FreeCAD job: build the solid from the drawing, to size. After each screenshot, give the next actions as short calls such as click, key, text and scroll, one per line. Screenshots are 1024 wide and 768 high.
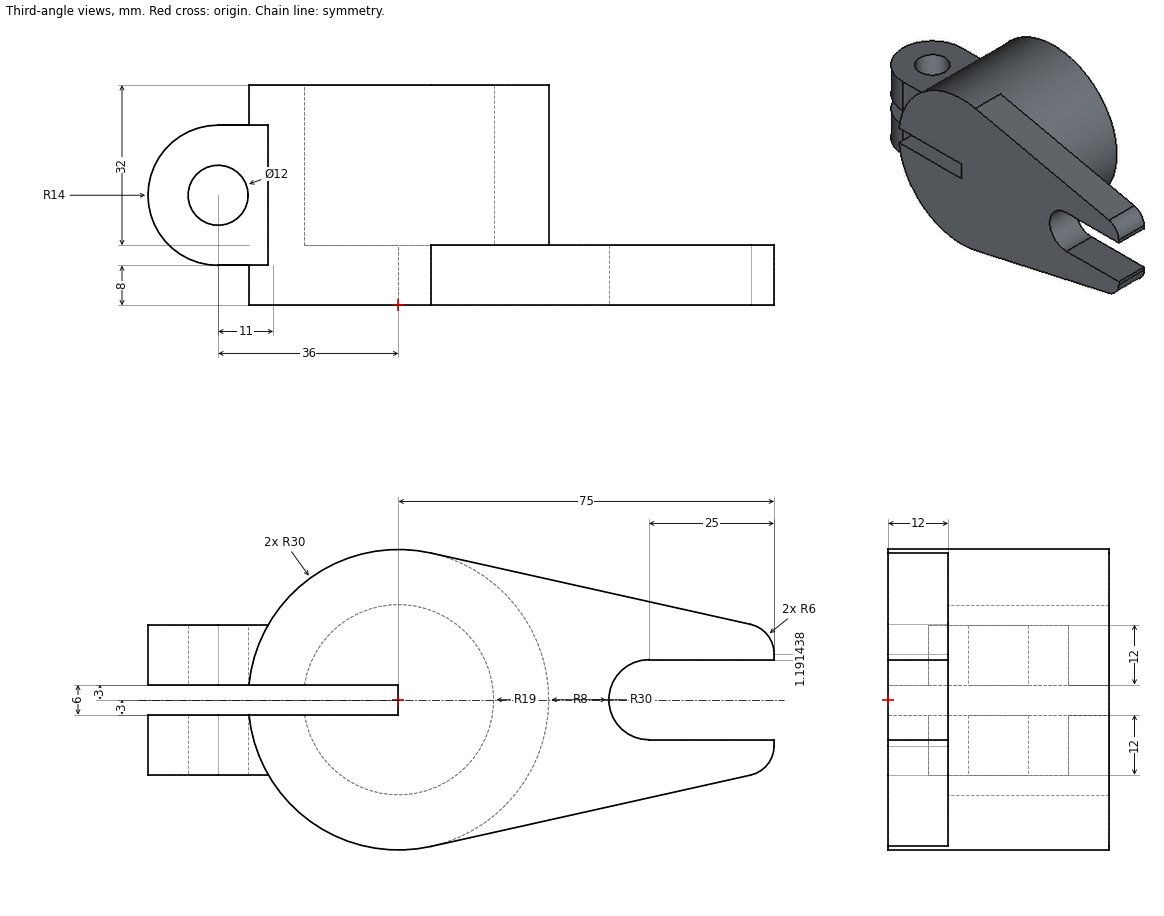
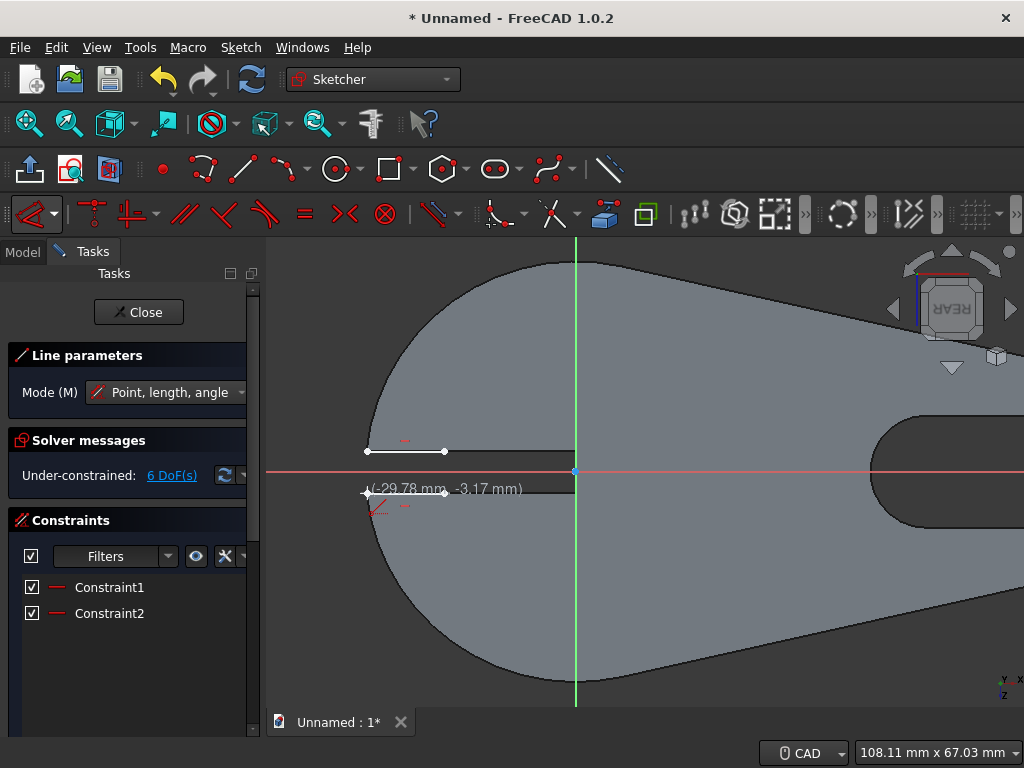
click(284, 170)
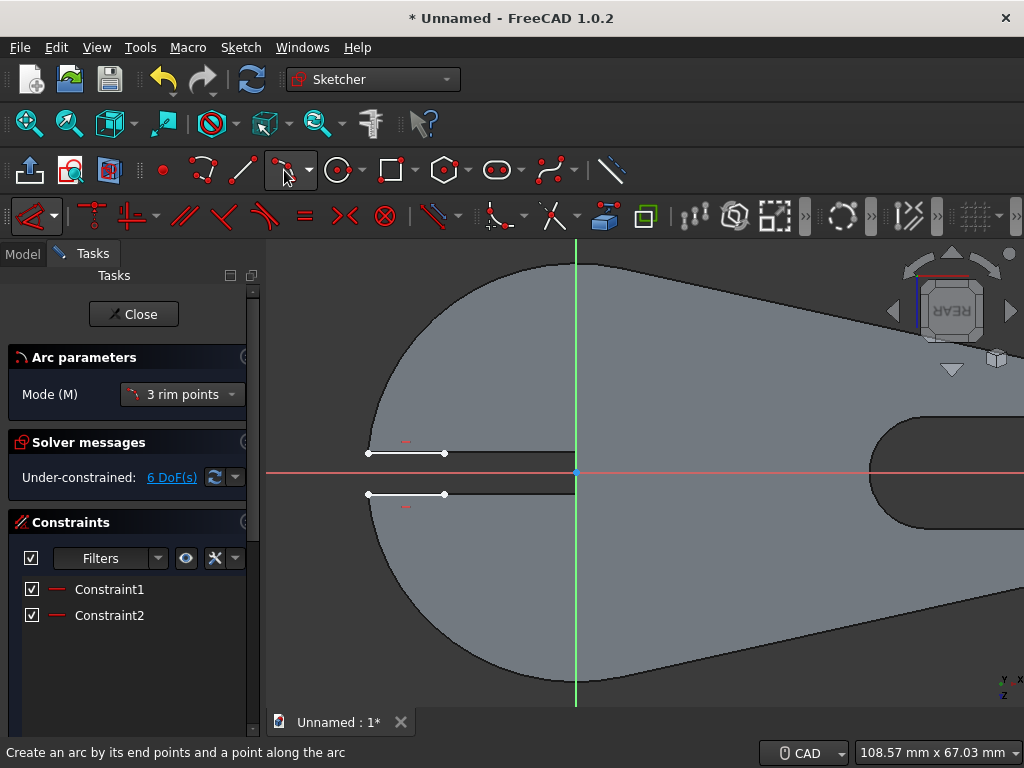
click(445, 453)
click(445, 495)
click(686, 547)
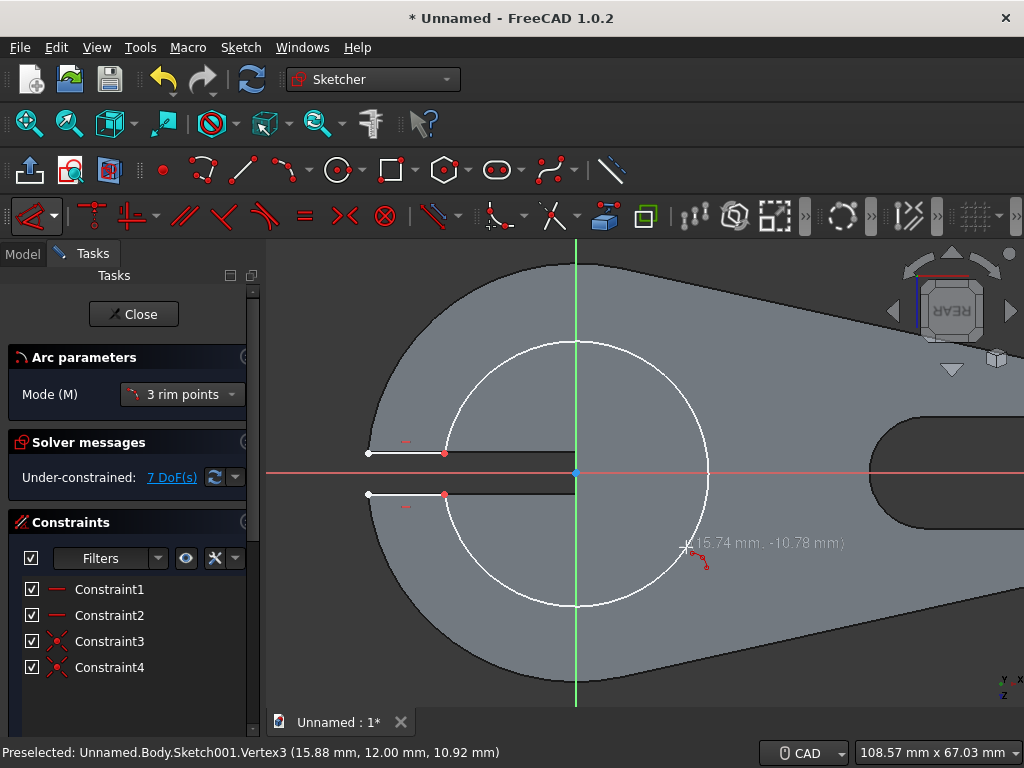
click(368, 495)
click(368, 453)
click(748, 592)
key(Escape)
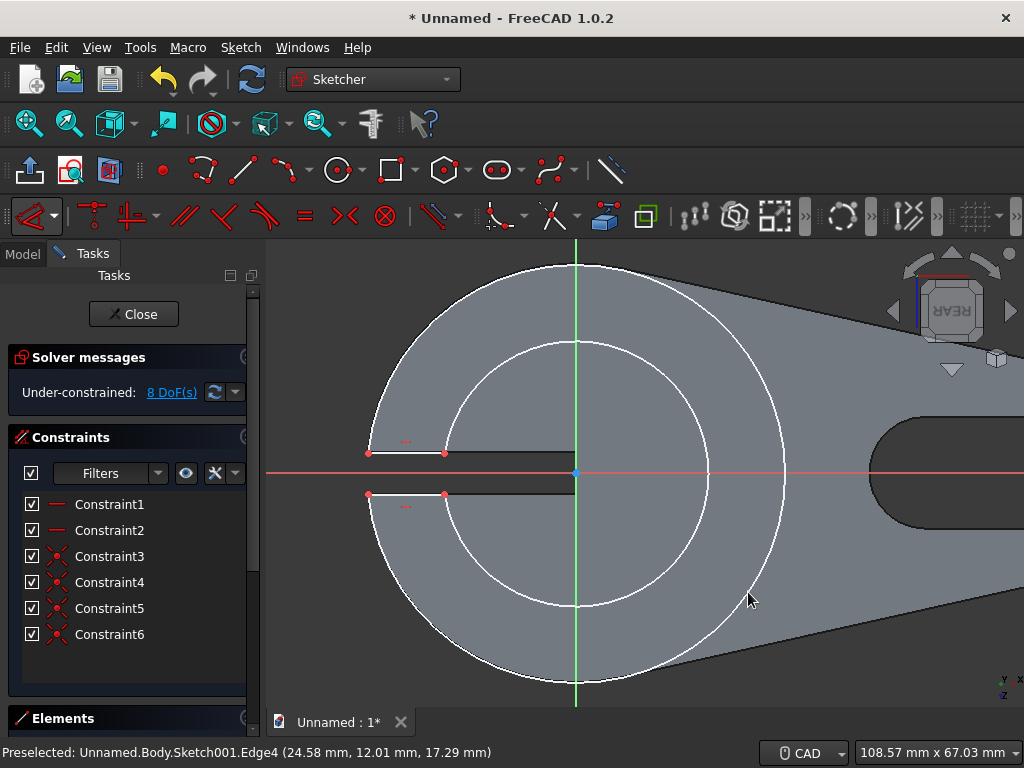
click(625, 597)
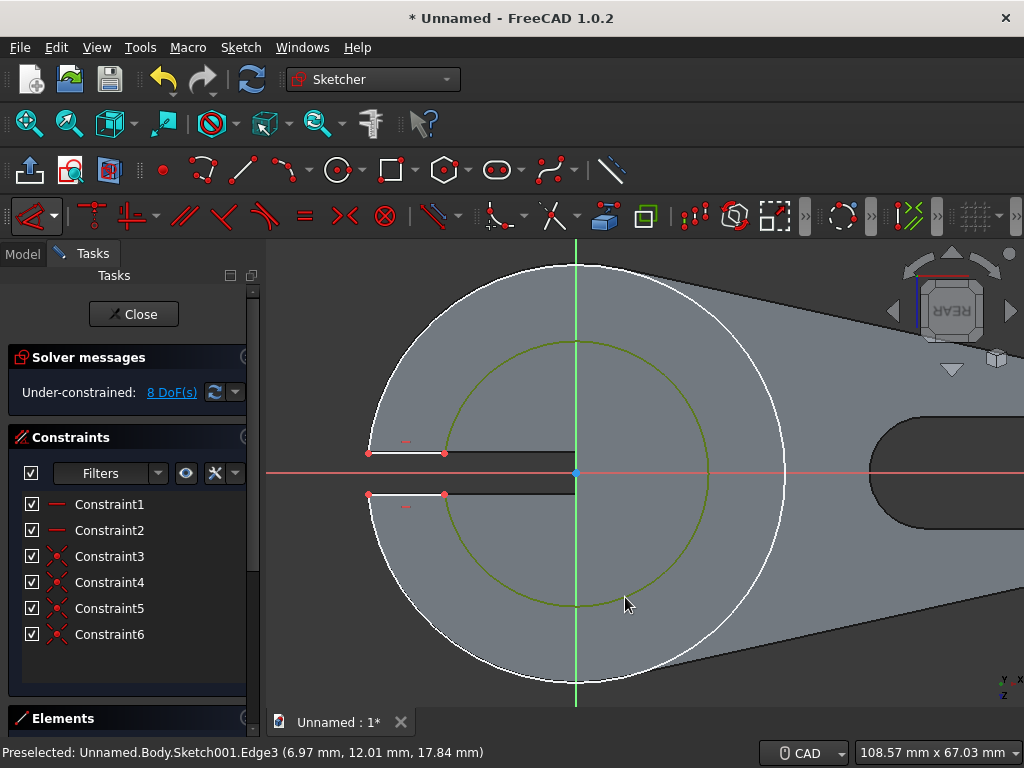
click(649, 670)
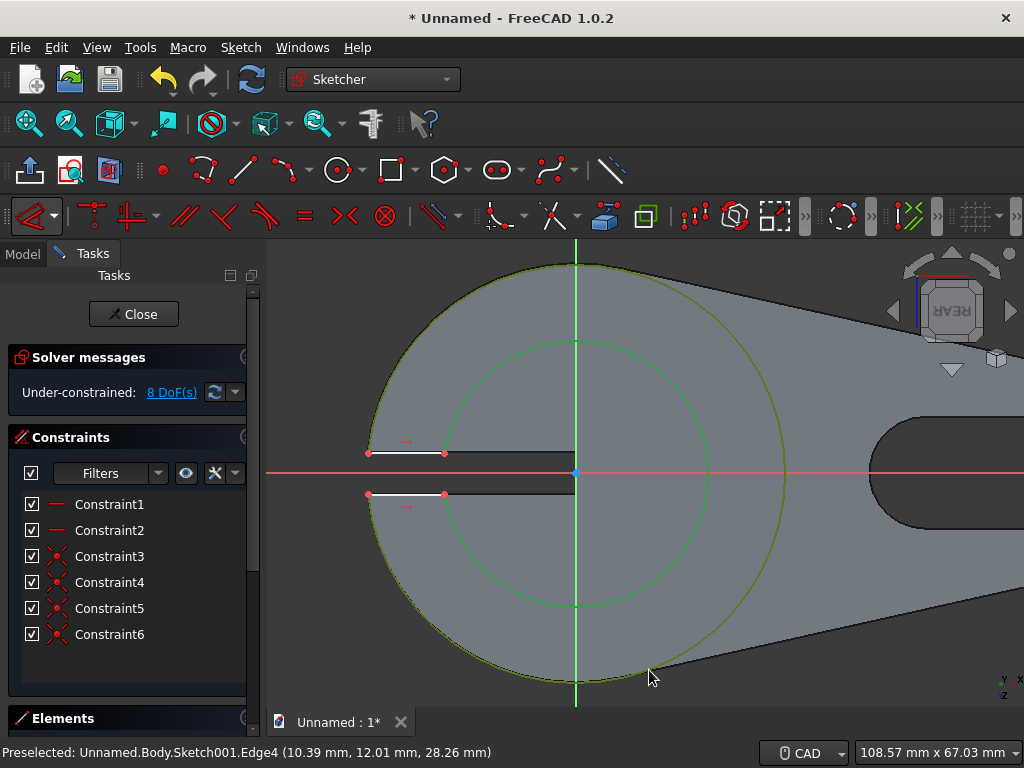
key(c)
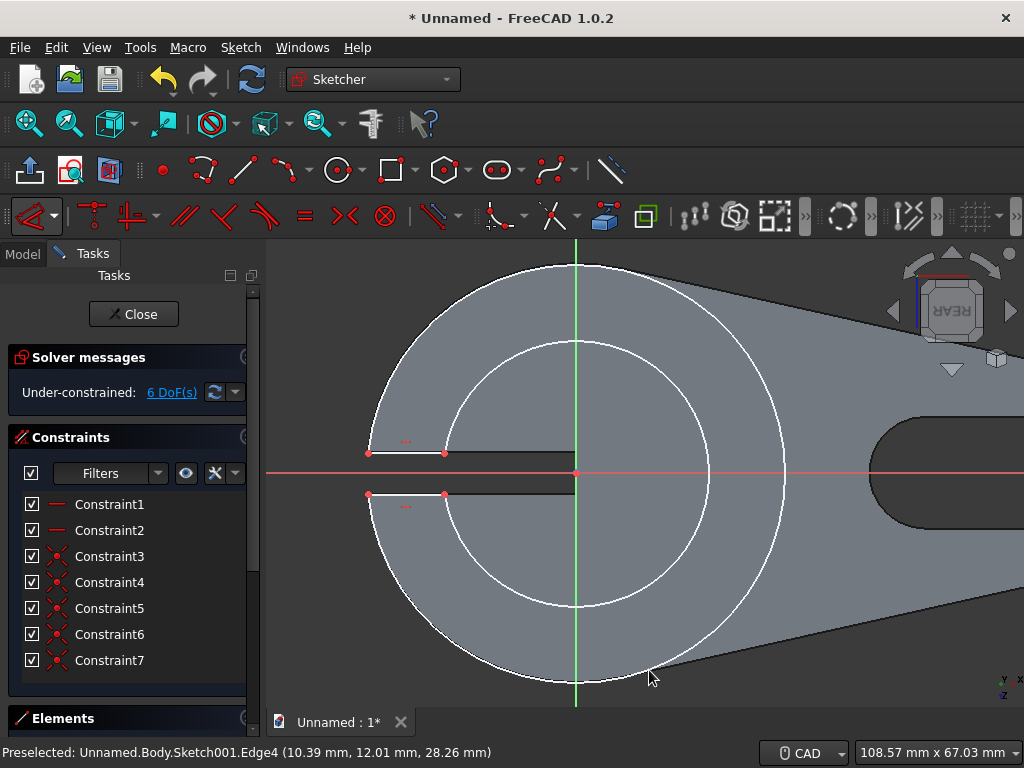
drag(566, 463, 586, 484)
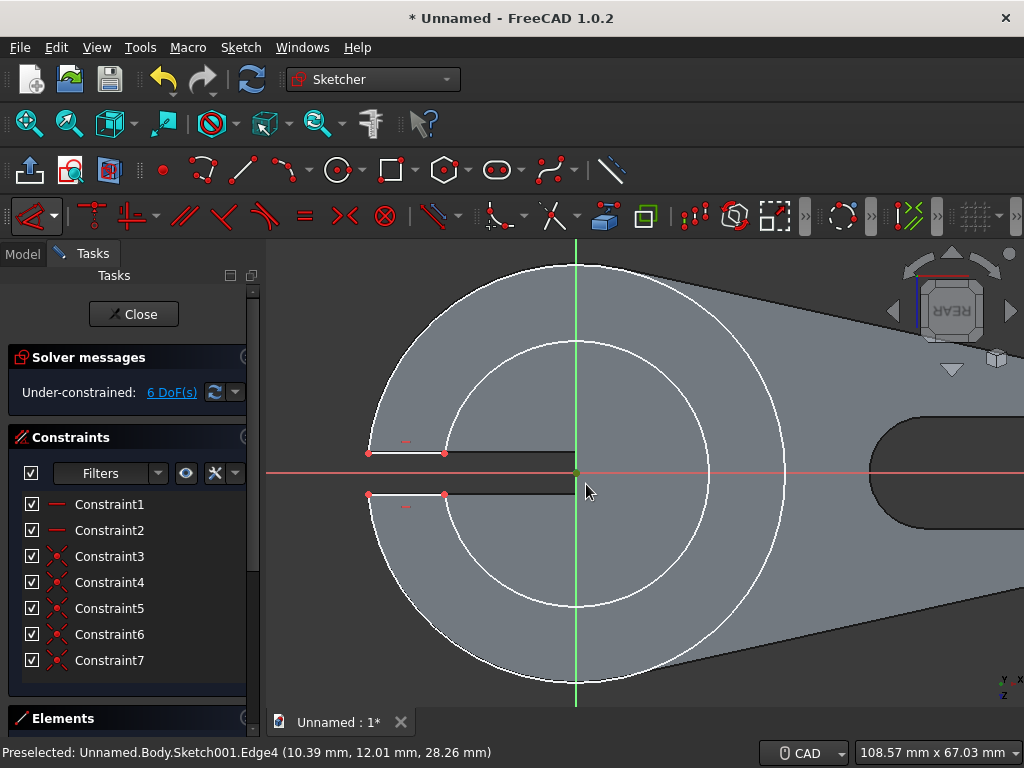
key(c)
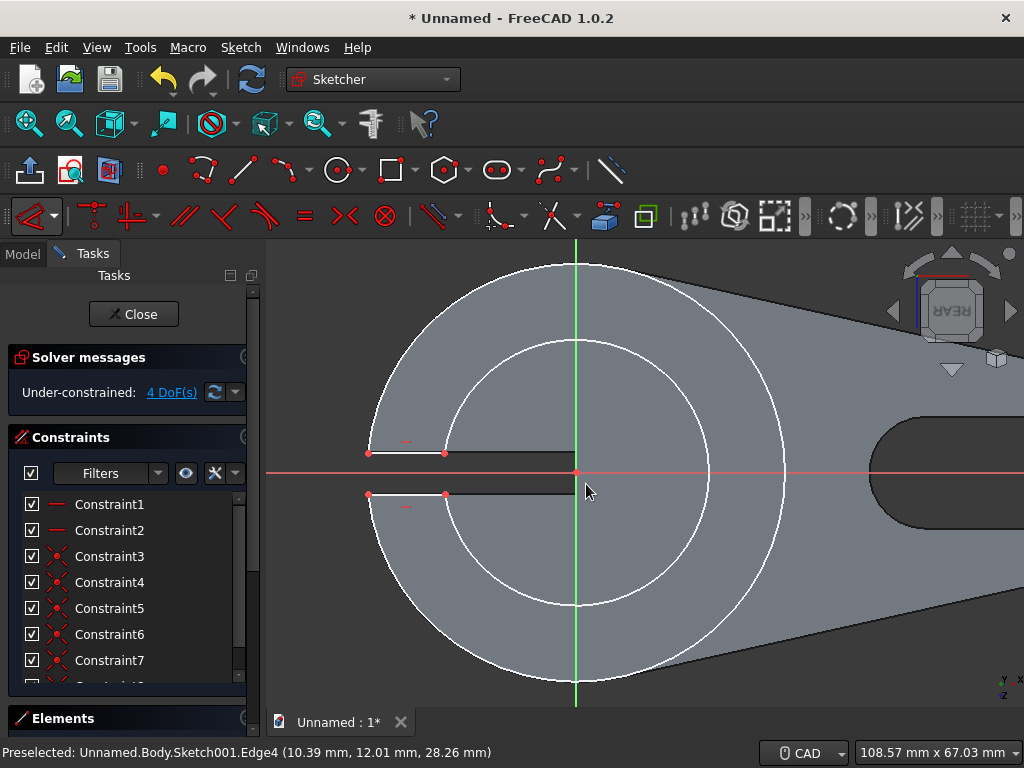
click(626, 596)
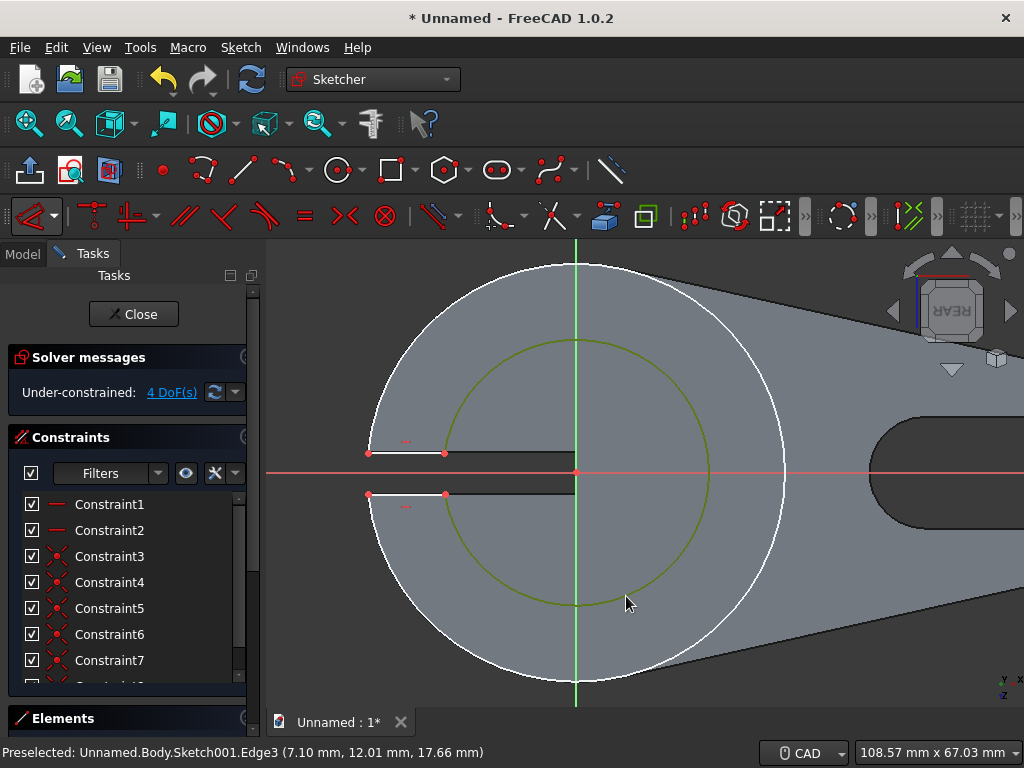
key(k)
key(r)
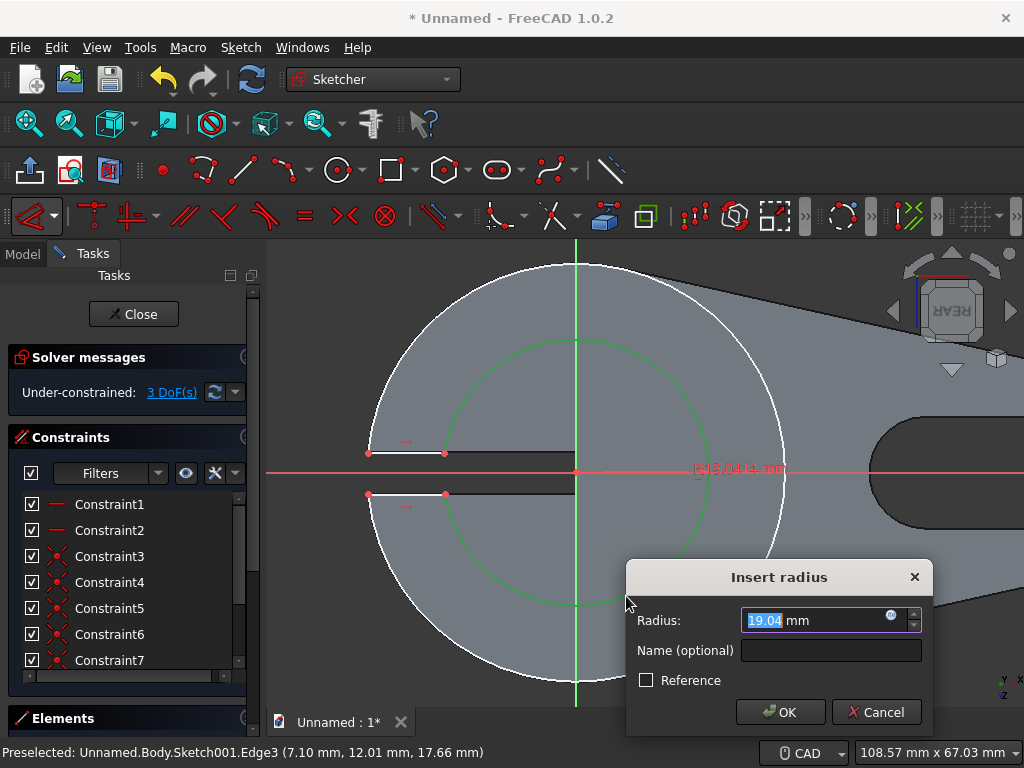
text(19)
key(Return)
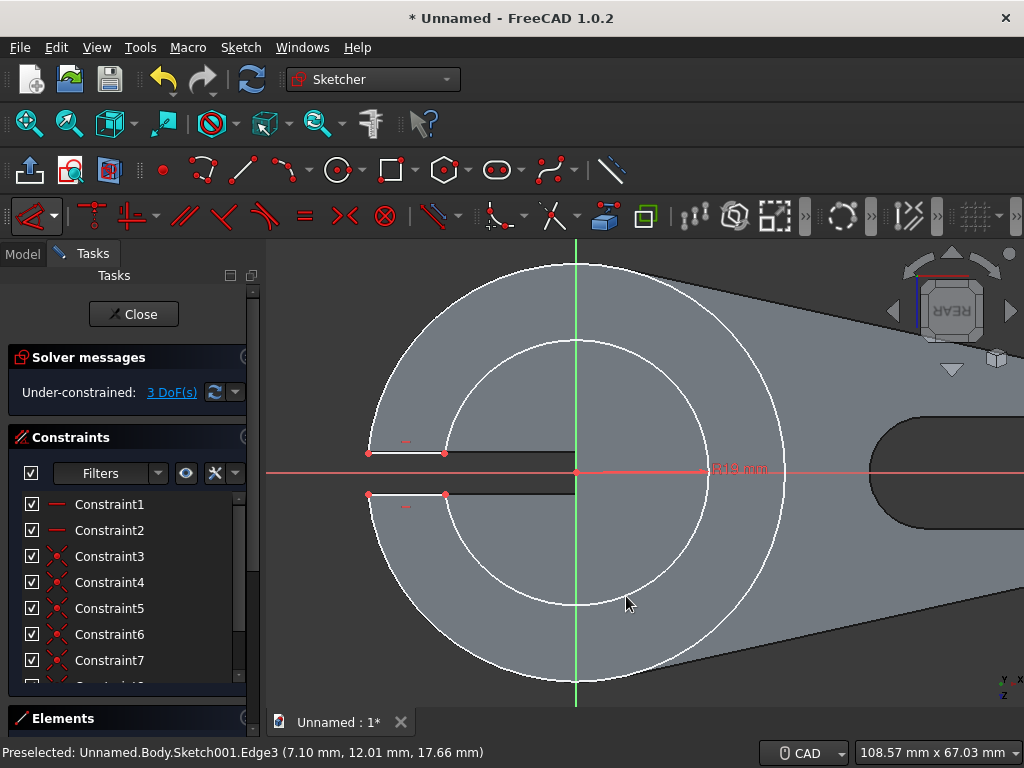
click(650, 668)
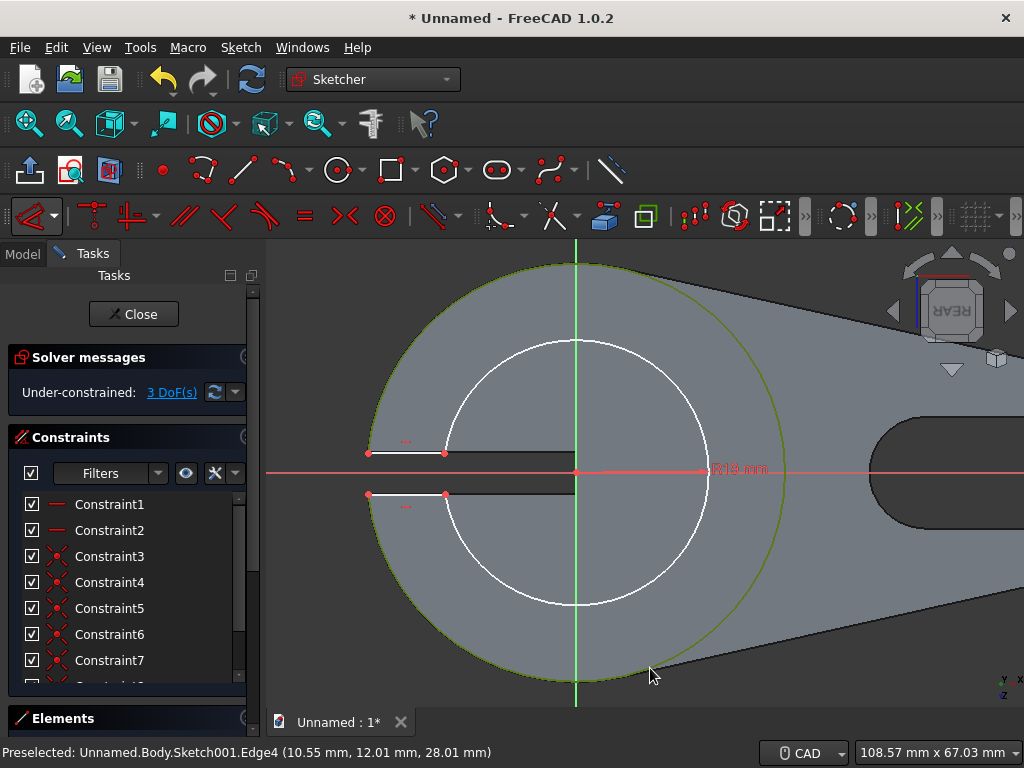
key(k)
key(r)